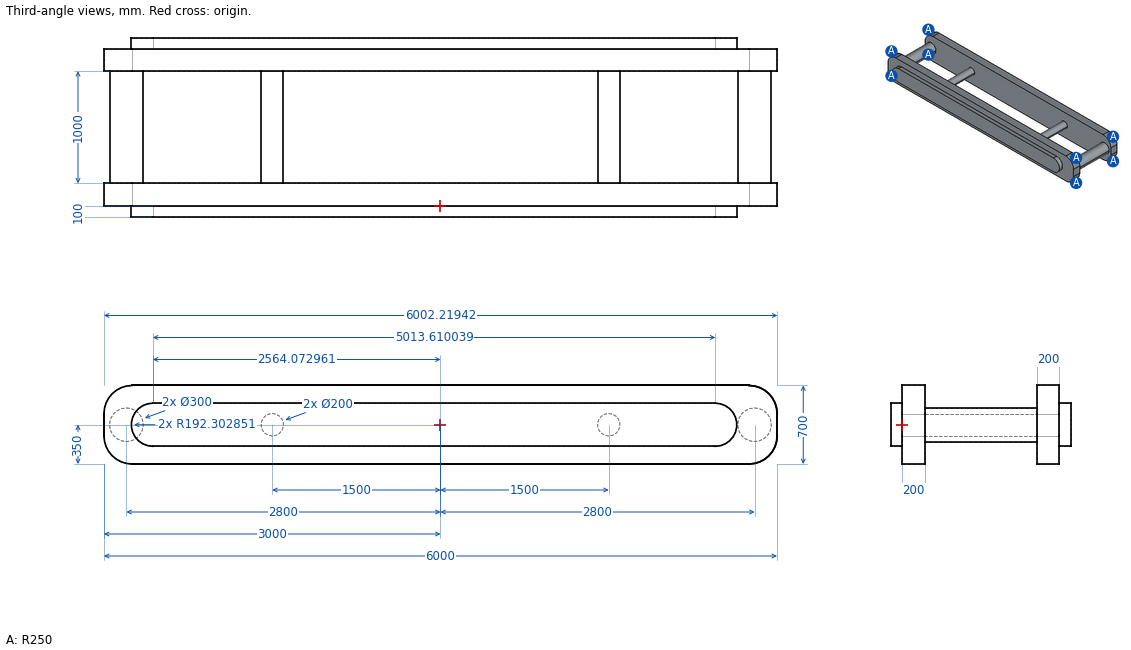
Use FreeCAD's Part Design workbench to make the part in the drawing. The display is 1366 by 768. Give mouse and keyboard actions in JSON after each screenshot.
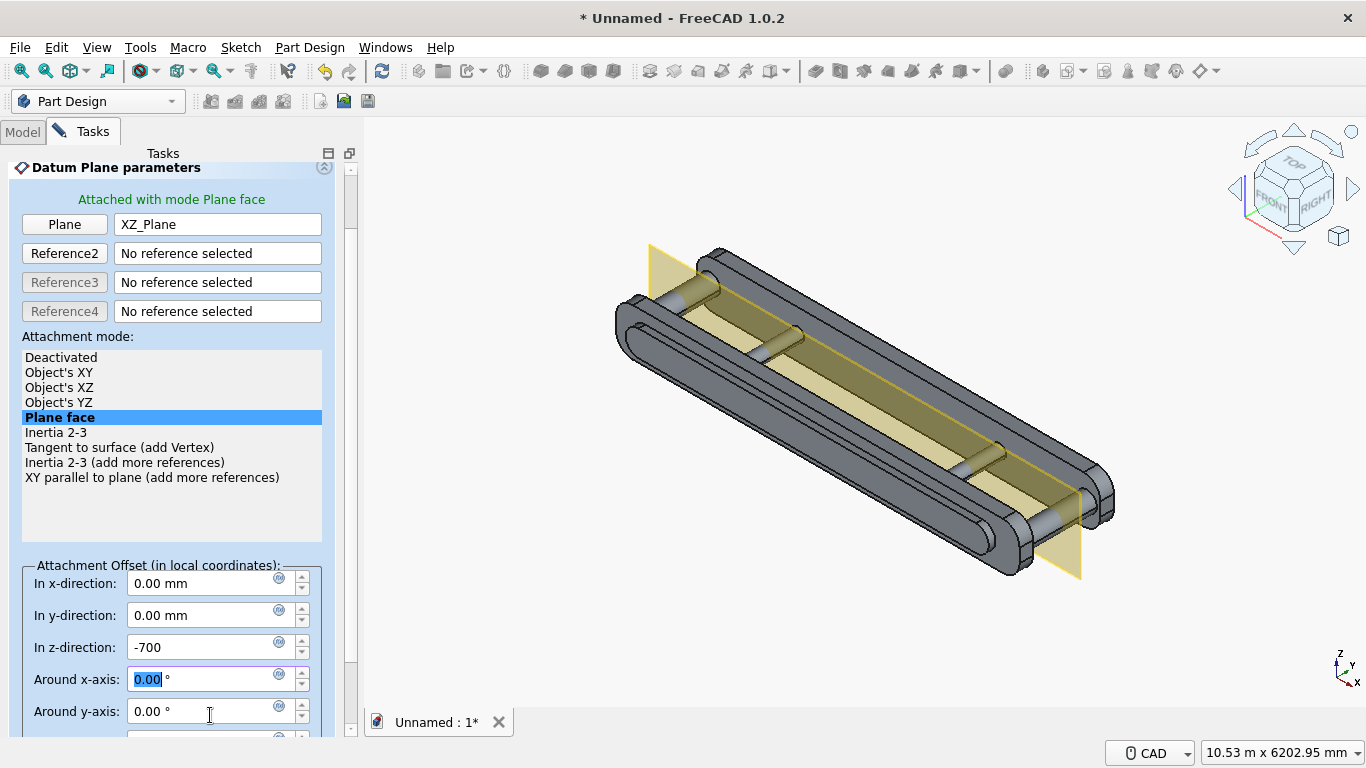
{"action": "scroll", "coordinate": [351, 450], "scroll_direction": "up", "scroll_amount": 2}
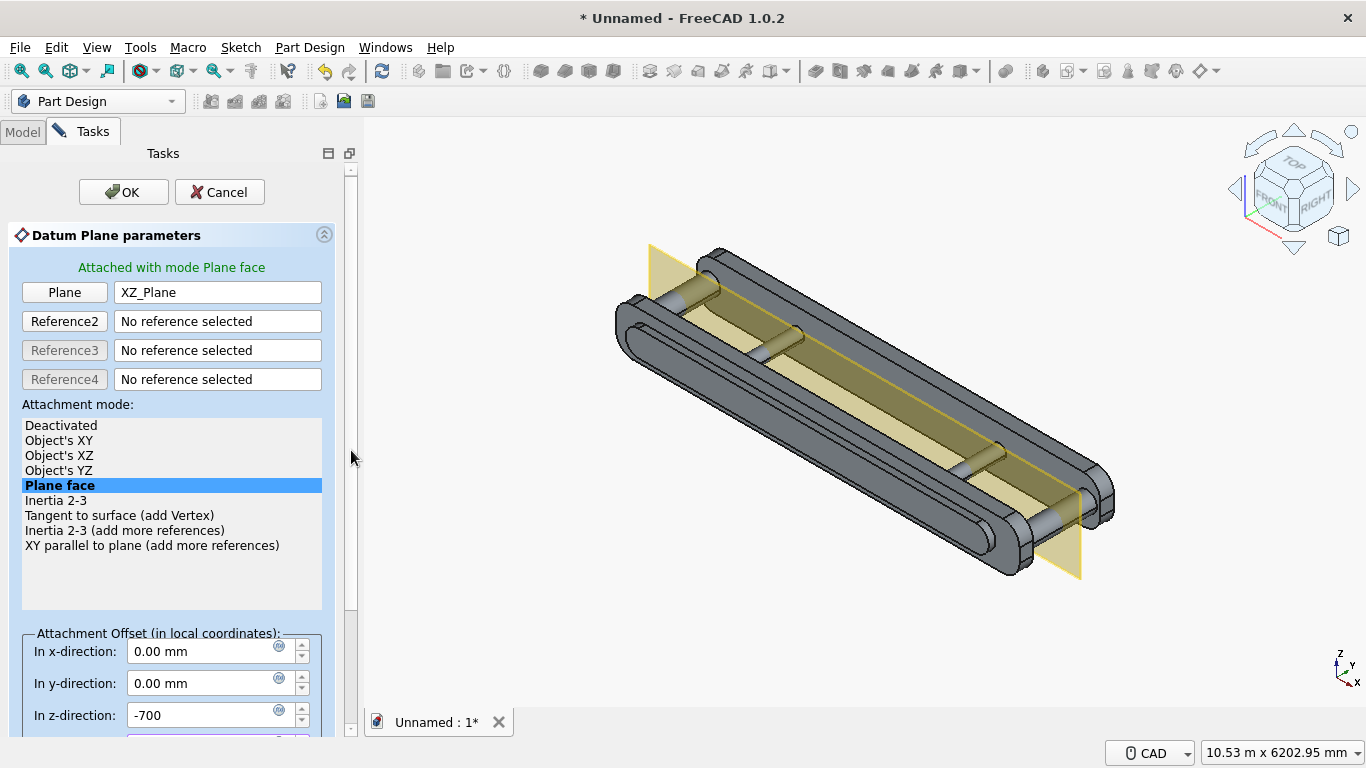
{"action": "left_click", "coordinate": [124, 192]}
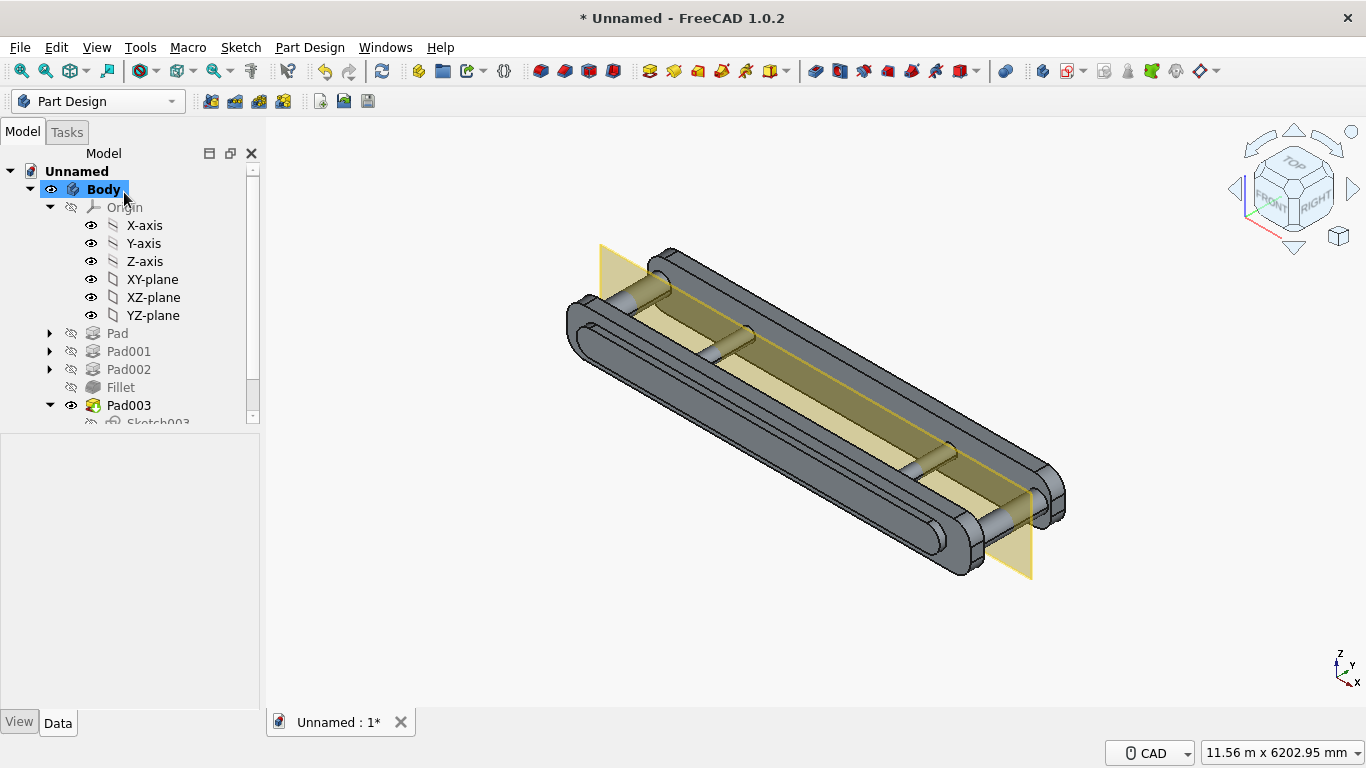
{"action": "left_click", "coordinate": [116, 405]}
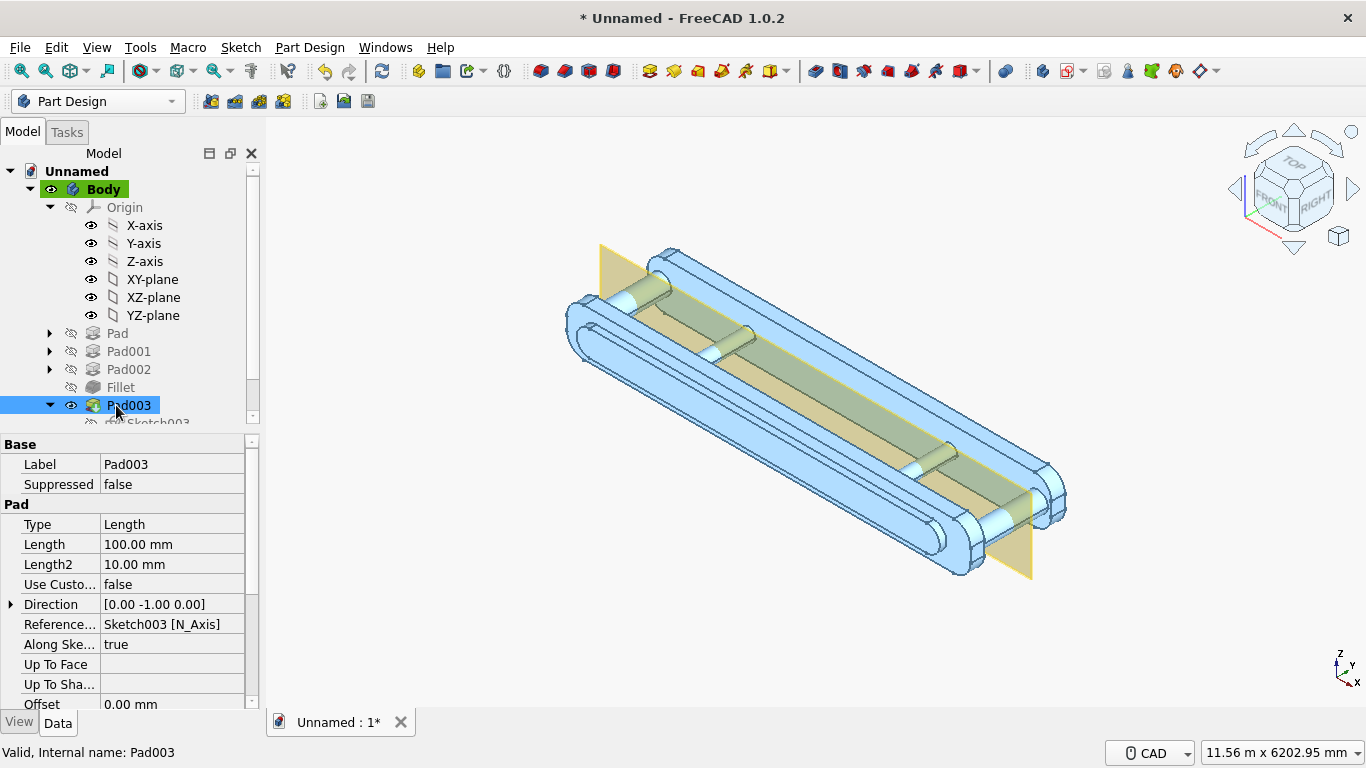
{"action": "left_click", "coordinate": [212, 102]}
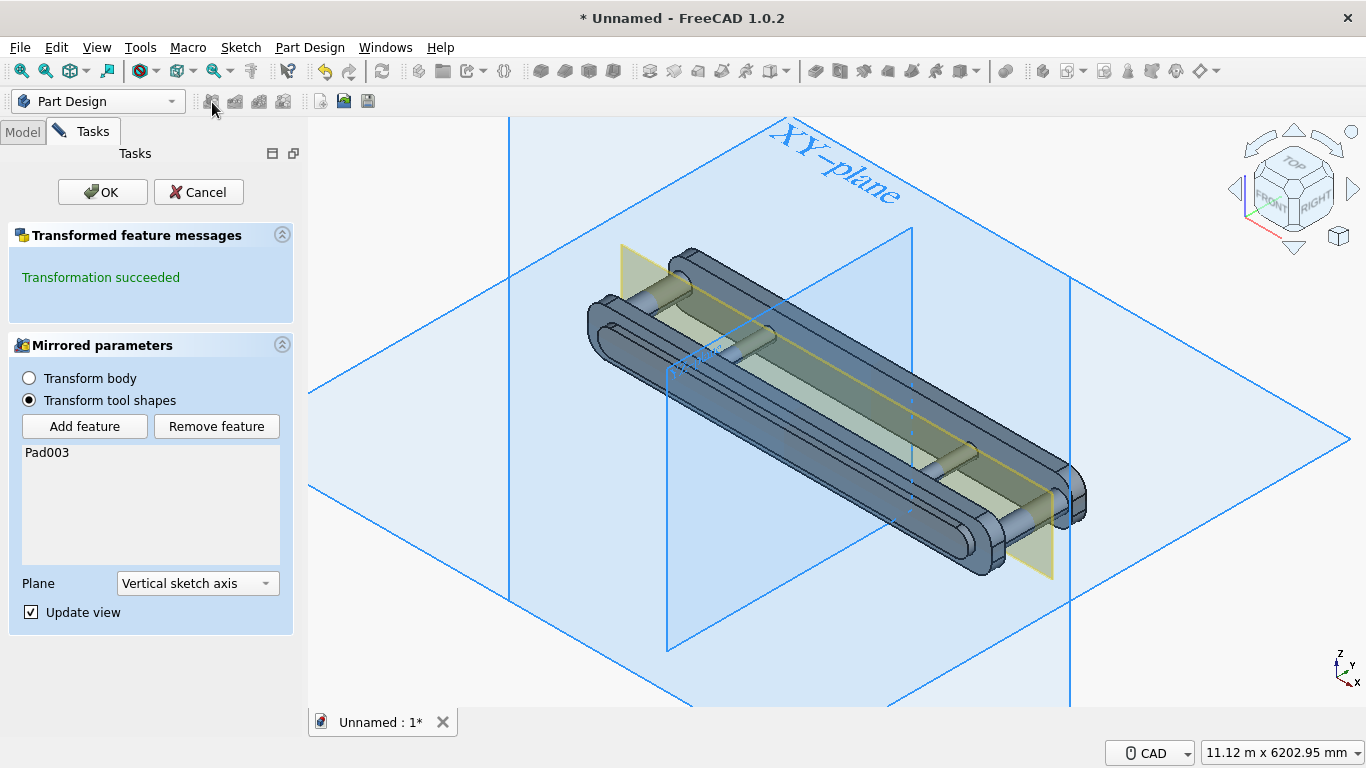
{"action": "left_click", "coordinate": [198, 584]}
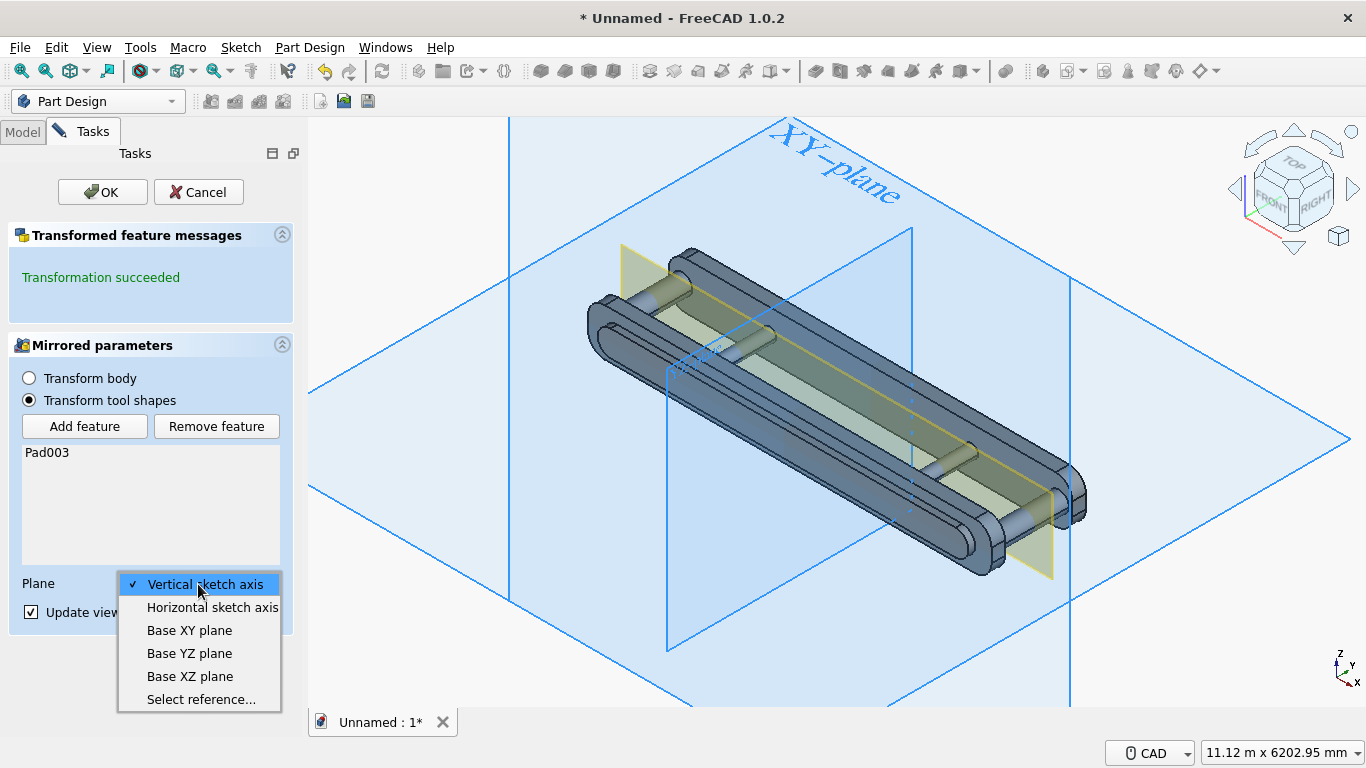
{"action": "left_click", "coordinate": [198, 700]}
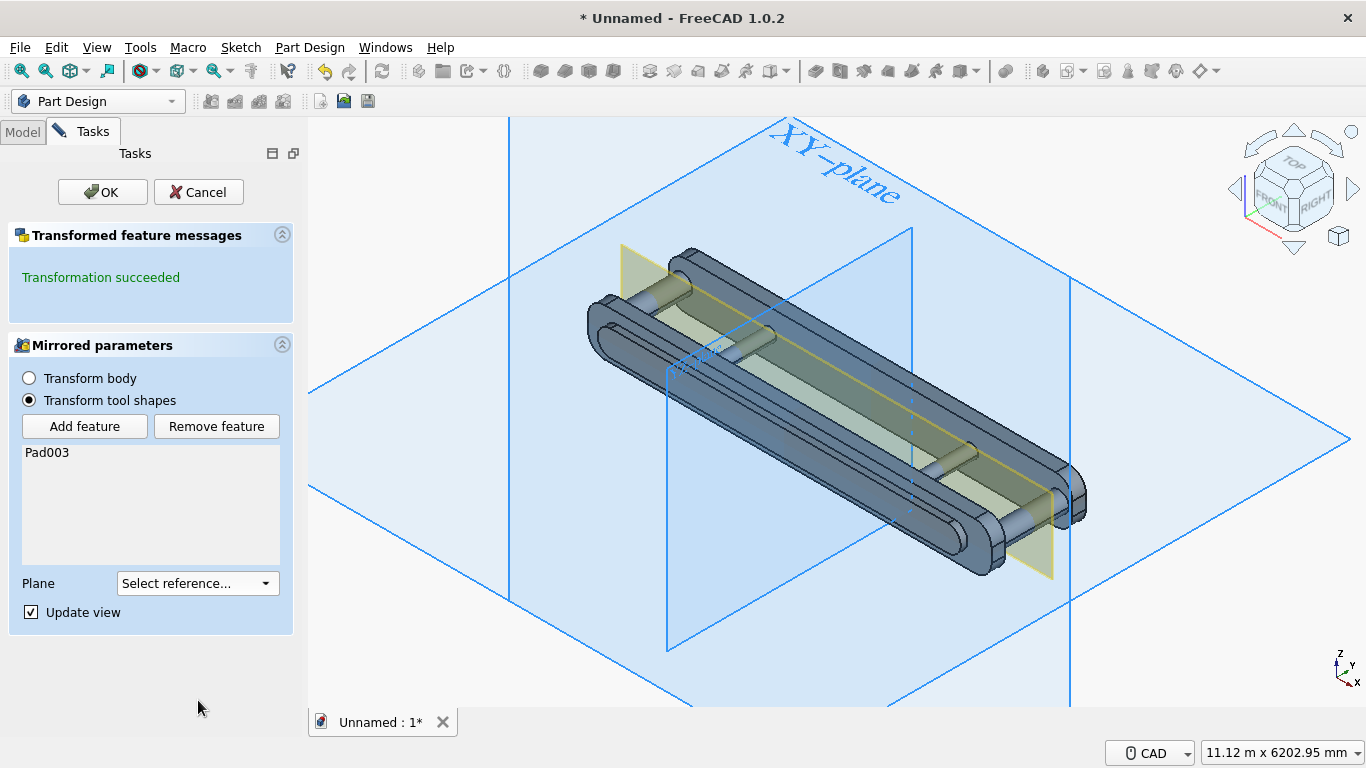
{"action": "left_click", "coordinate": [23, 131]}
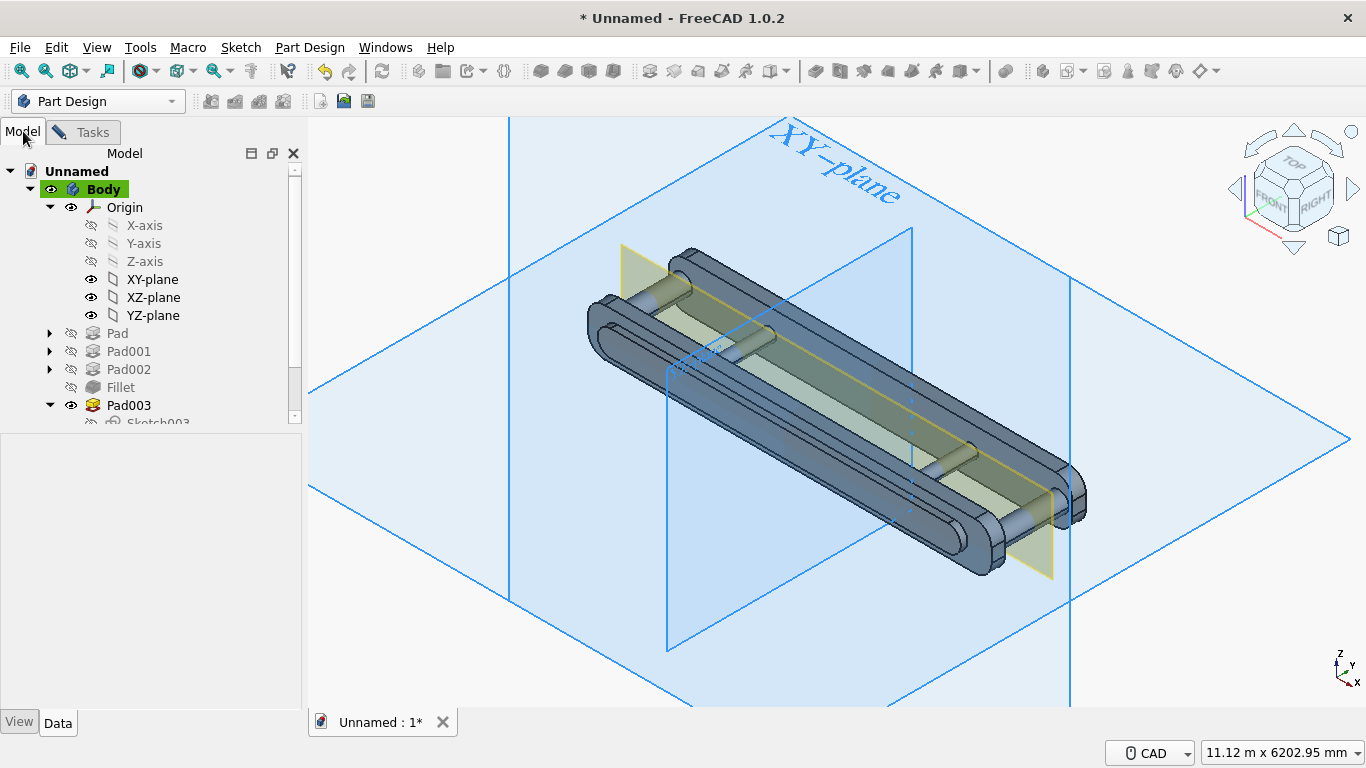
{"action": "scroll", "coordinate": [100, 293], "scroll_direction": "down", "scroll_amount": 3}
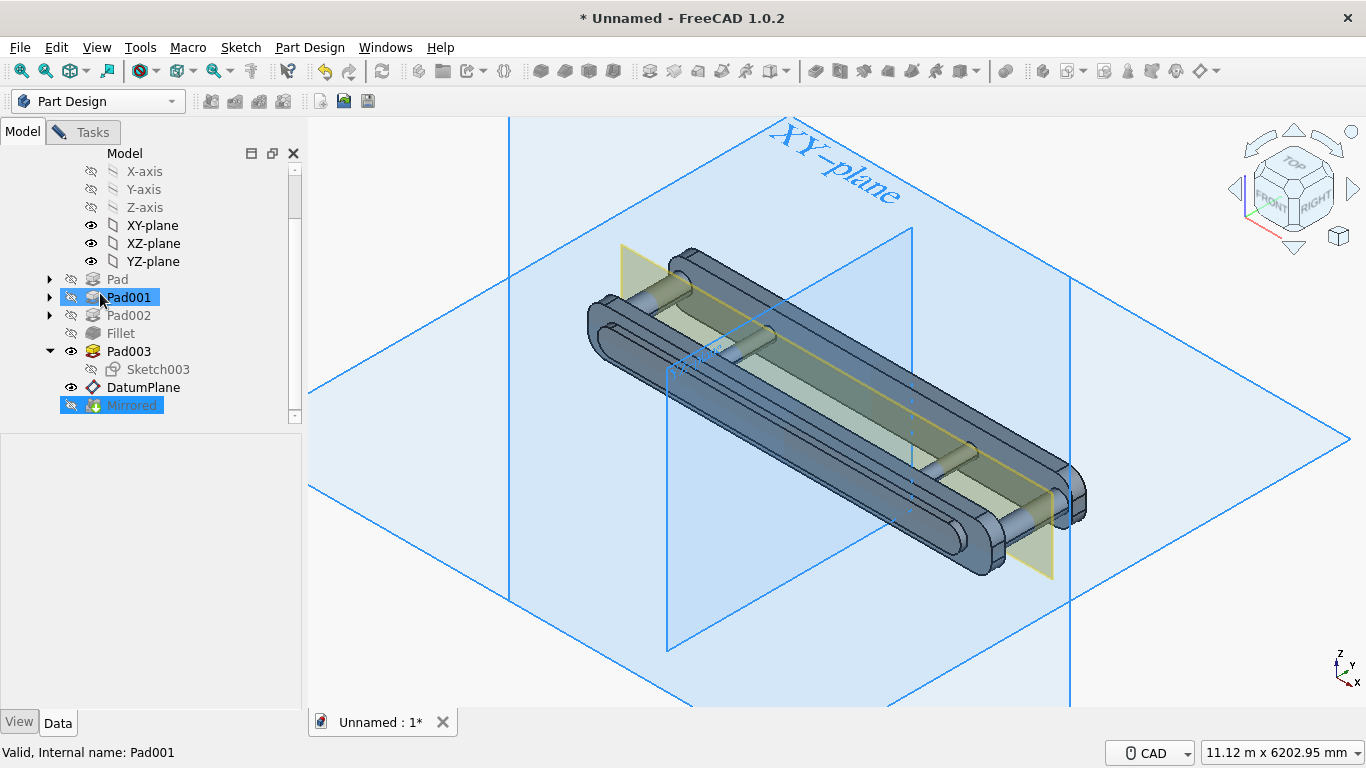
{"action": "left_click", "coordinate": [116, 387]}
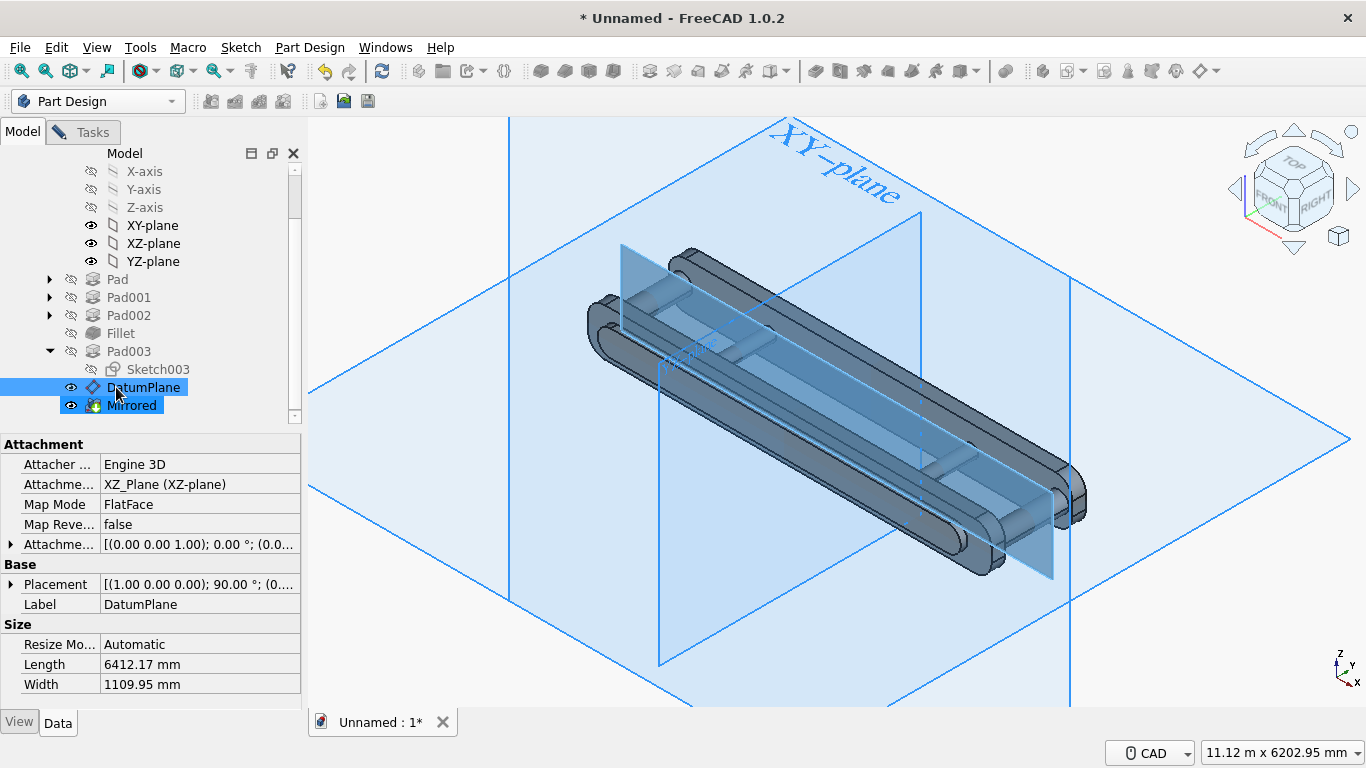
{"action": "left_click", "coordinate": [84, 131]}